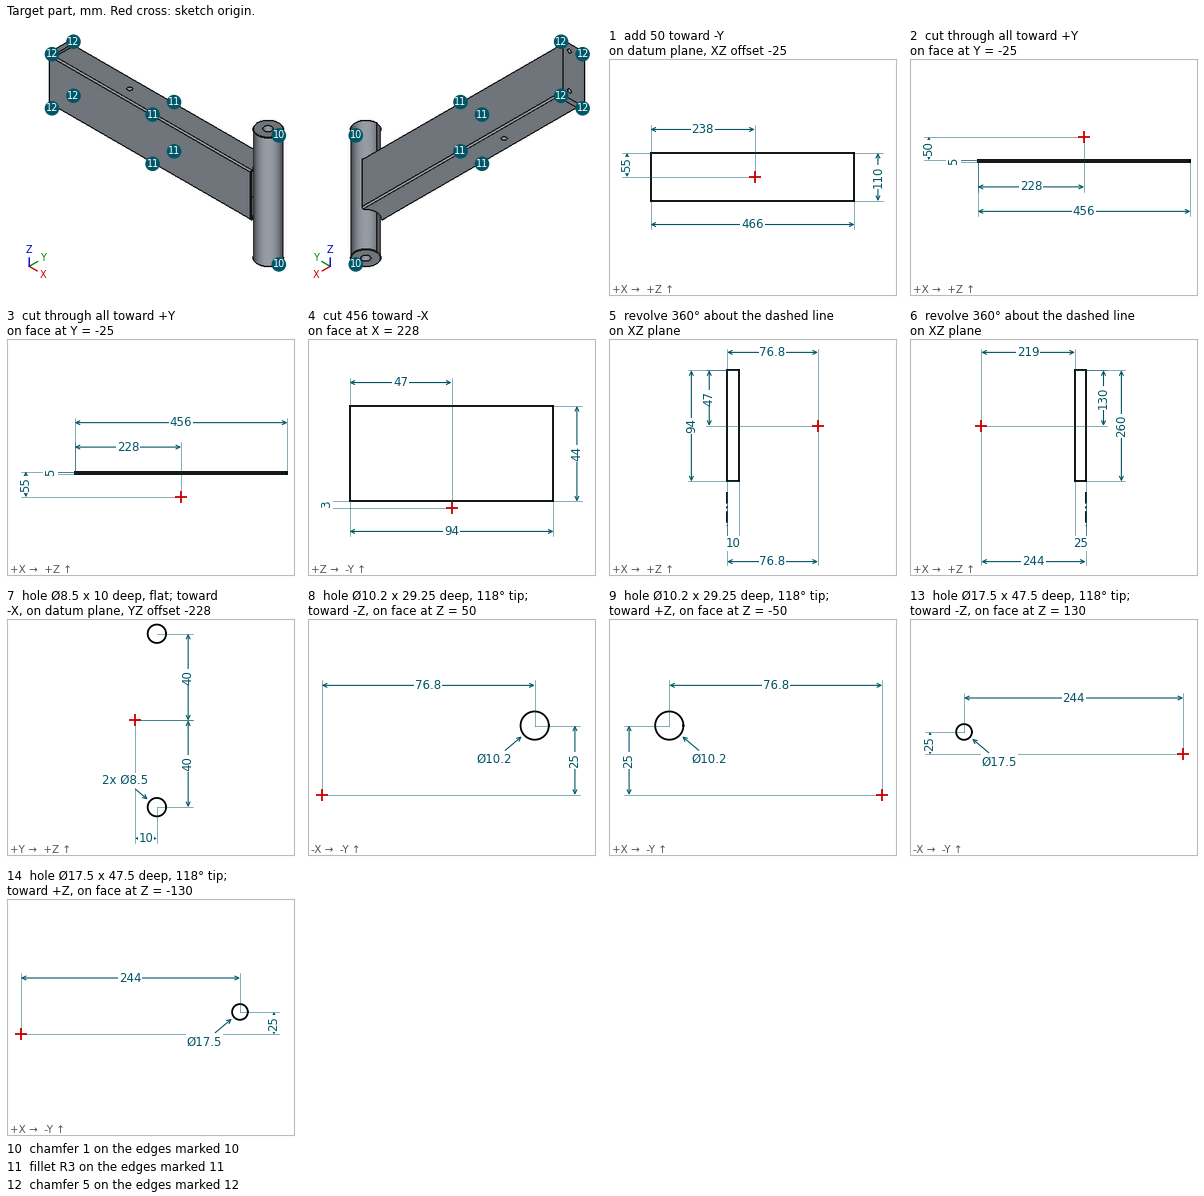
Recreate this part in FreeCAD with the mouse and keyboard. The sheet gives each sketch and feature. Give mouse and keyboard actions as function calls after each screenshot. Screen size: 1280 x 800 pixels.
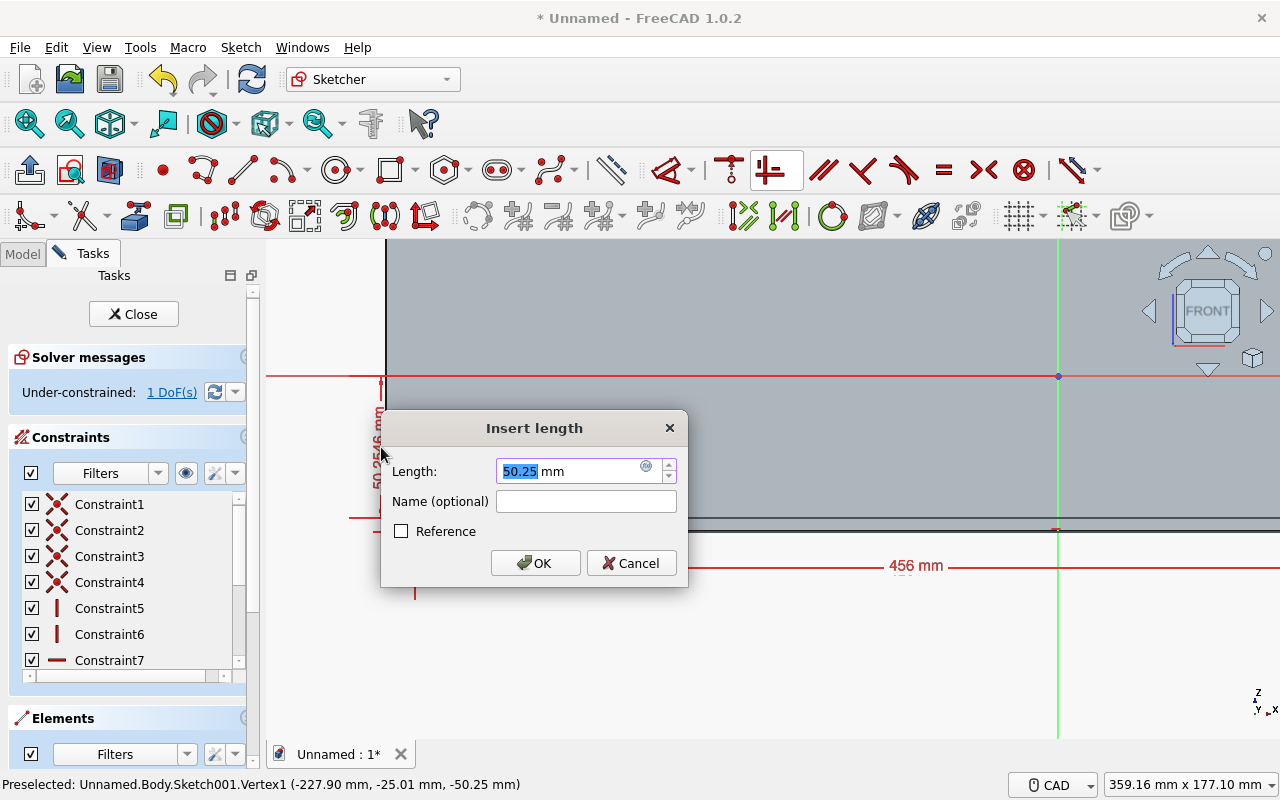
text(50)
key(Return)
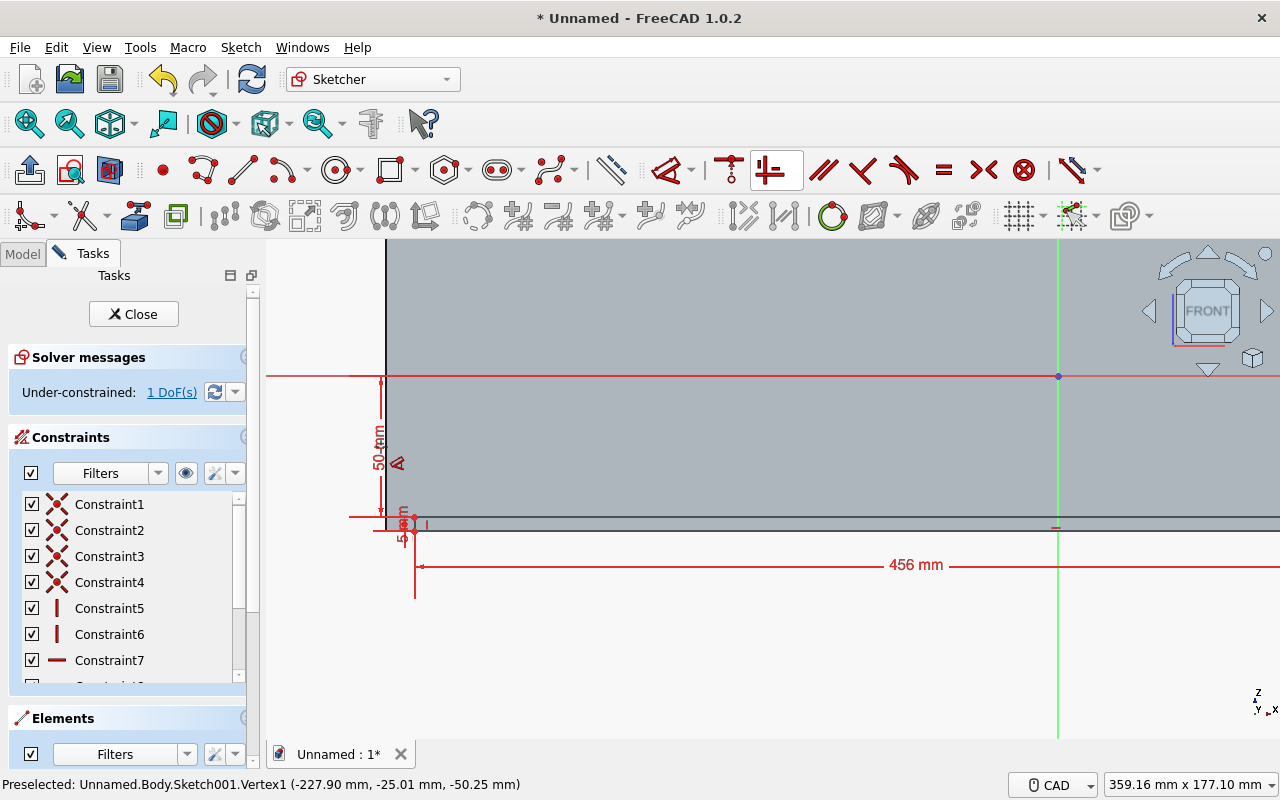
click(415, 517)
click(737, 342)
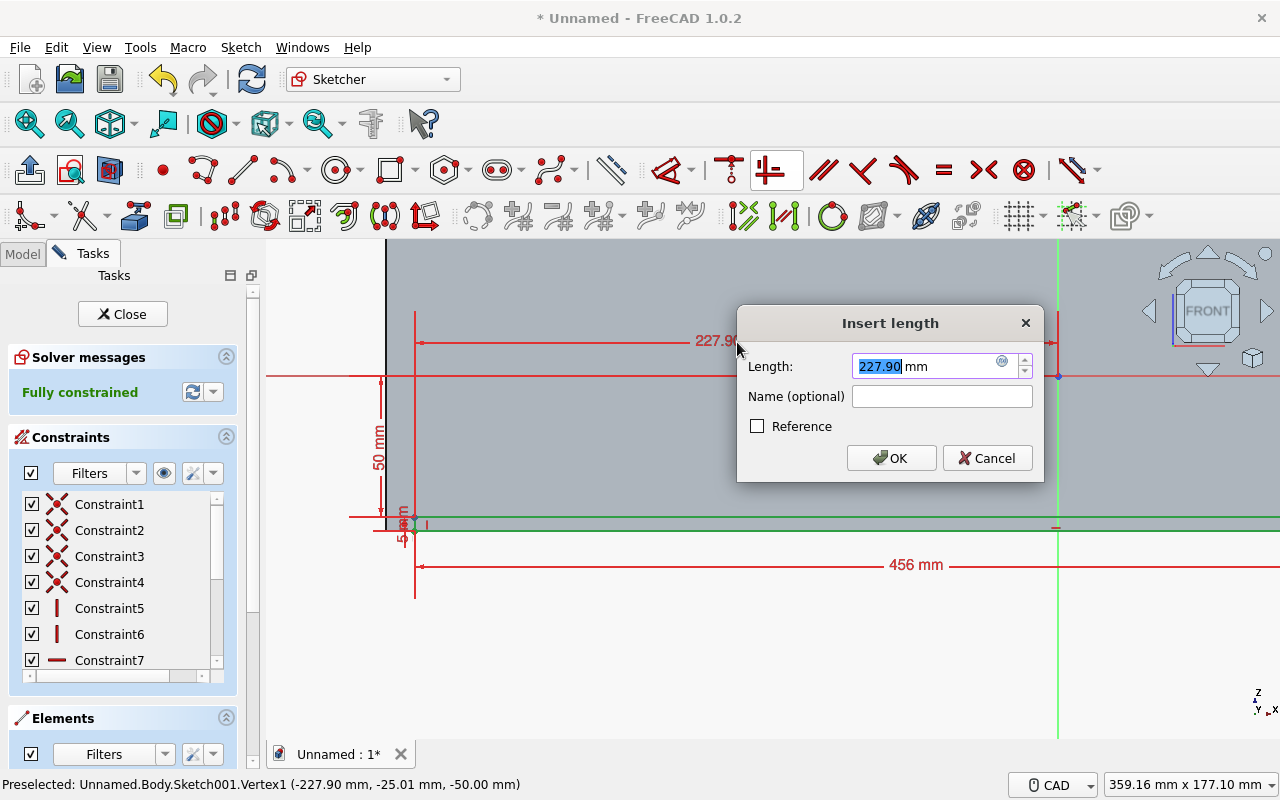
text(228)
key(Return)
key(Escape)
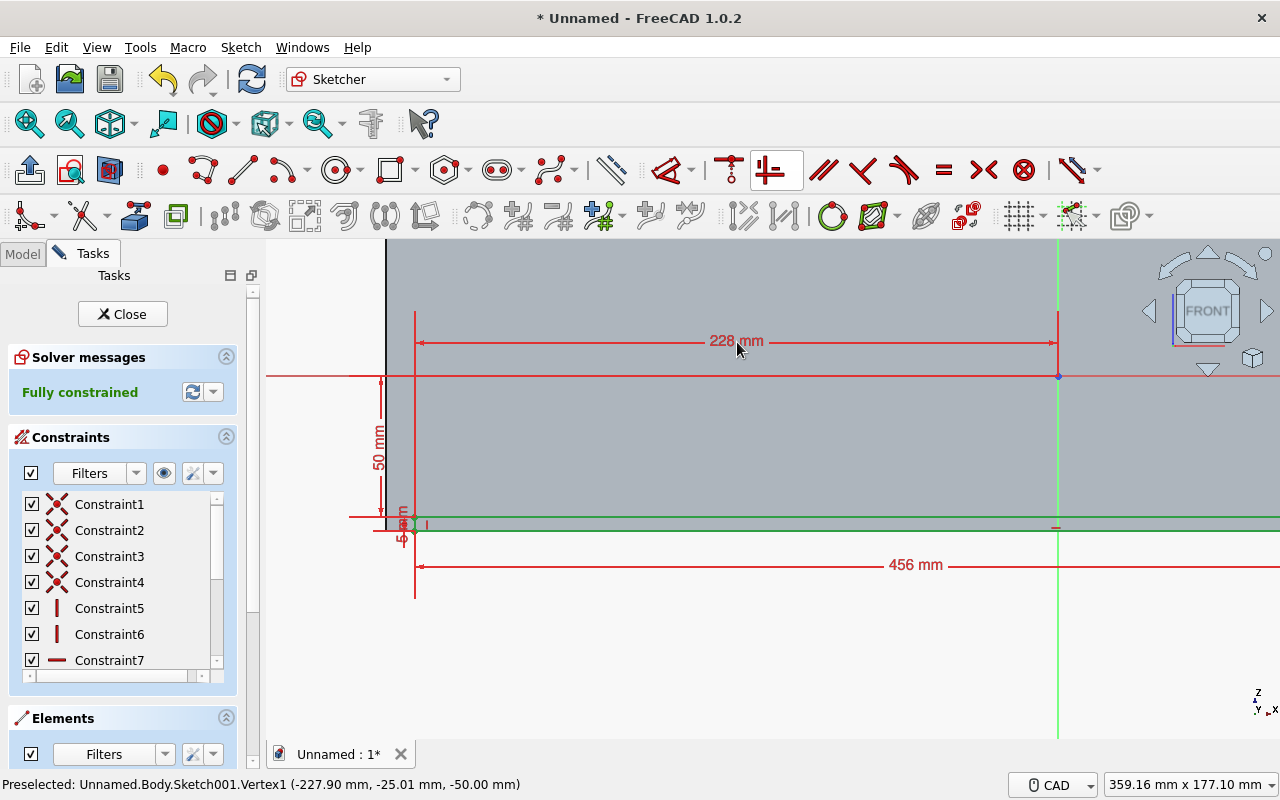
click(123, 314)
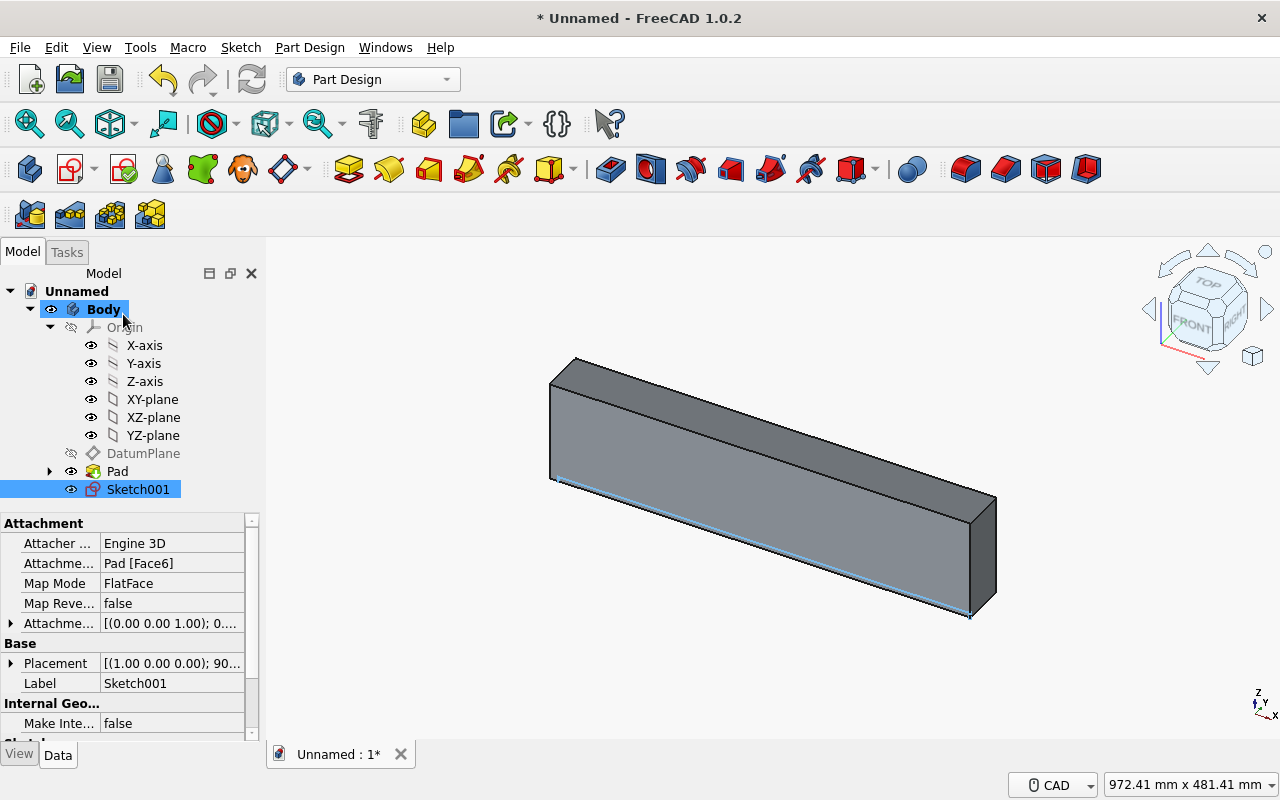
click(612, 170)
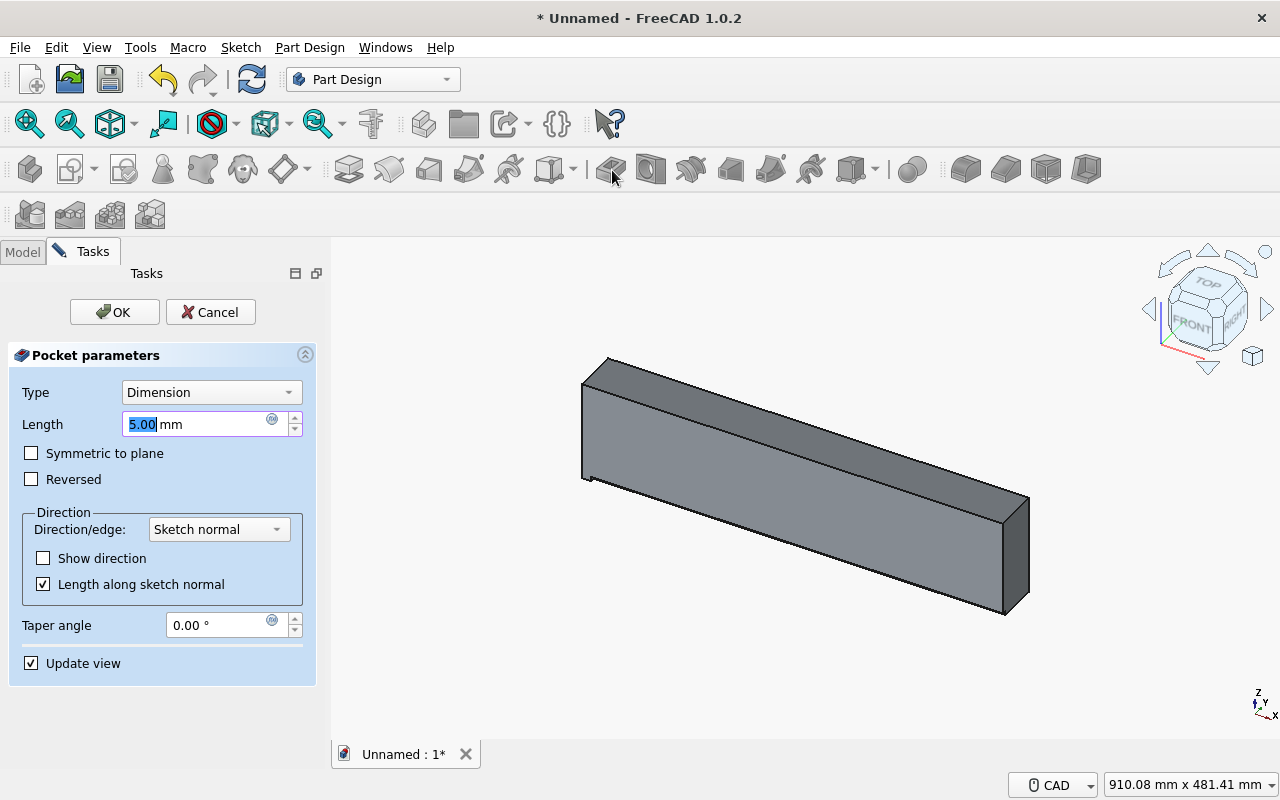
click(212, 392)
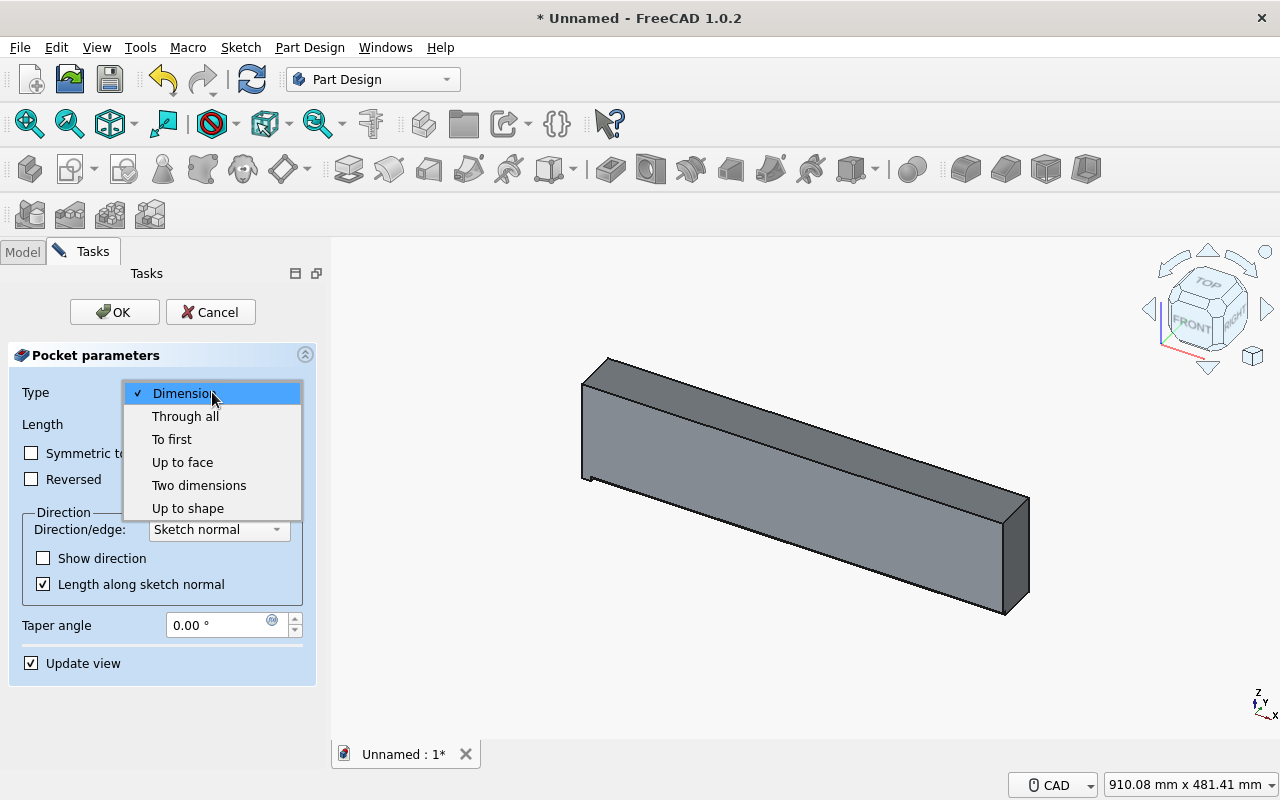
click(212, 416)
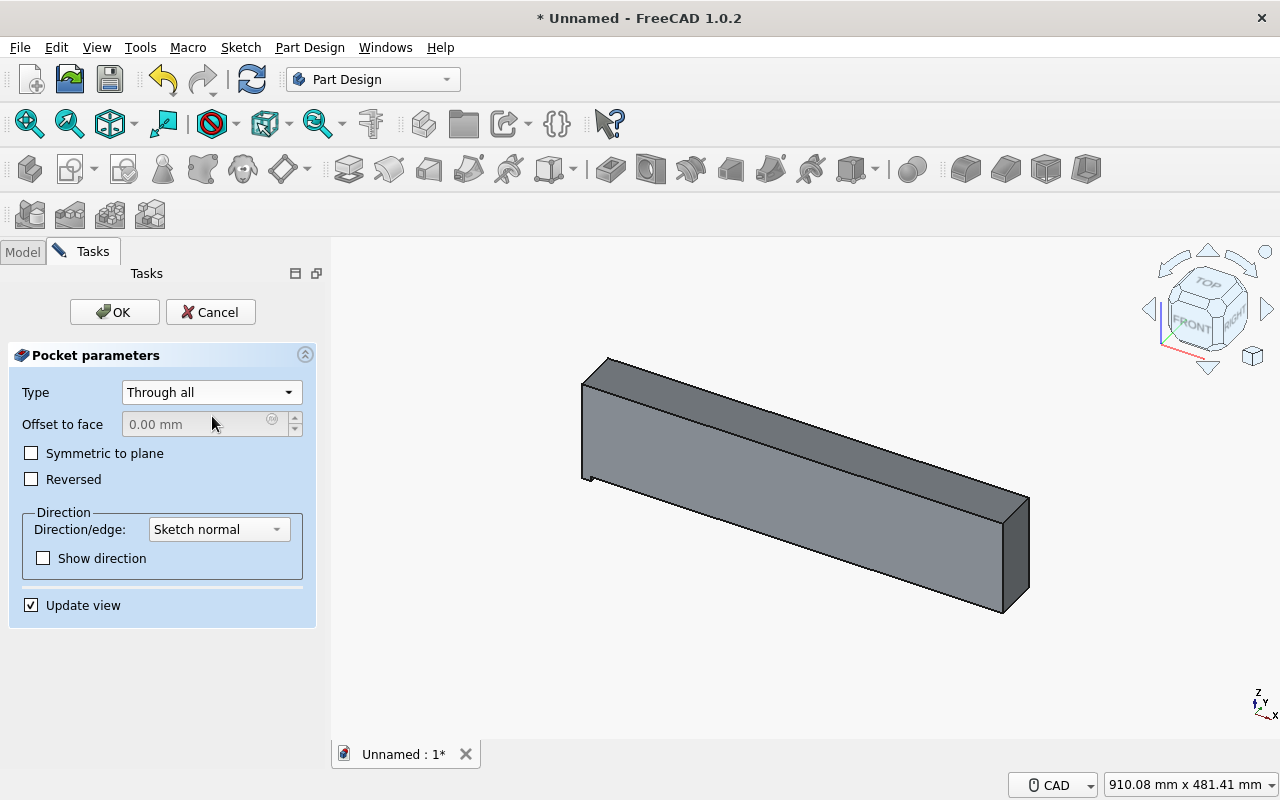
click(115, 312)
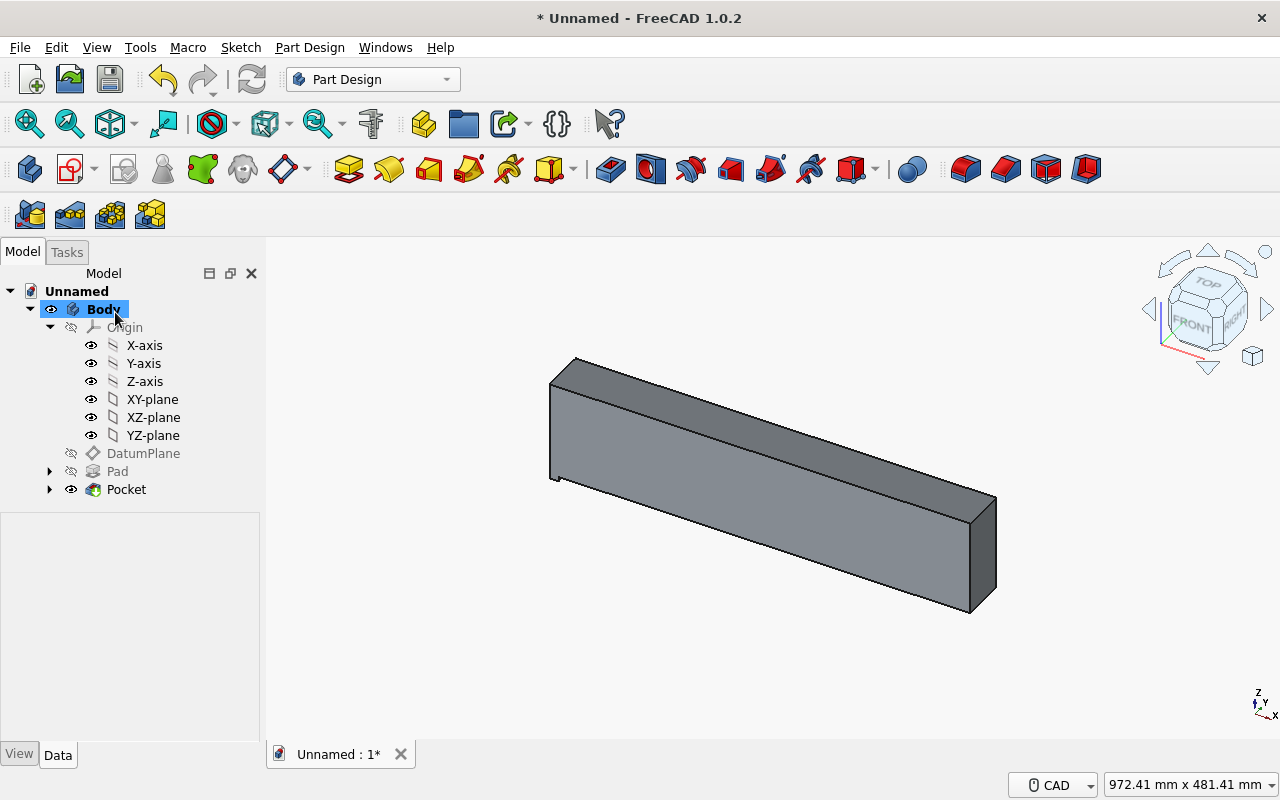
click(880, 540)